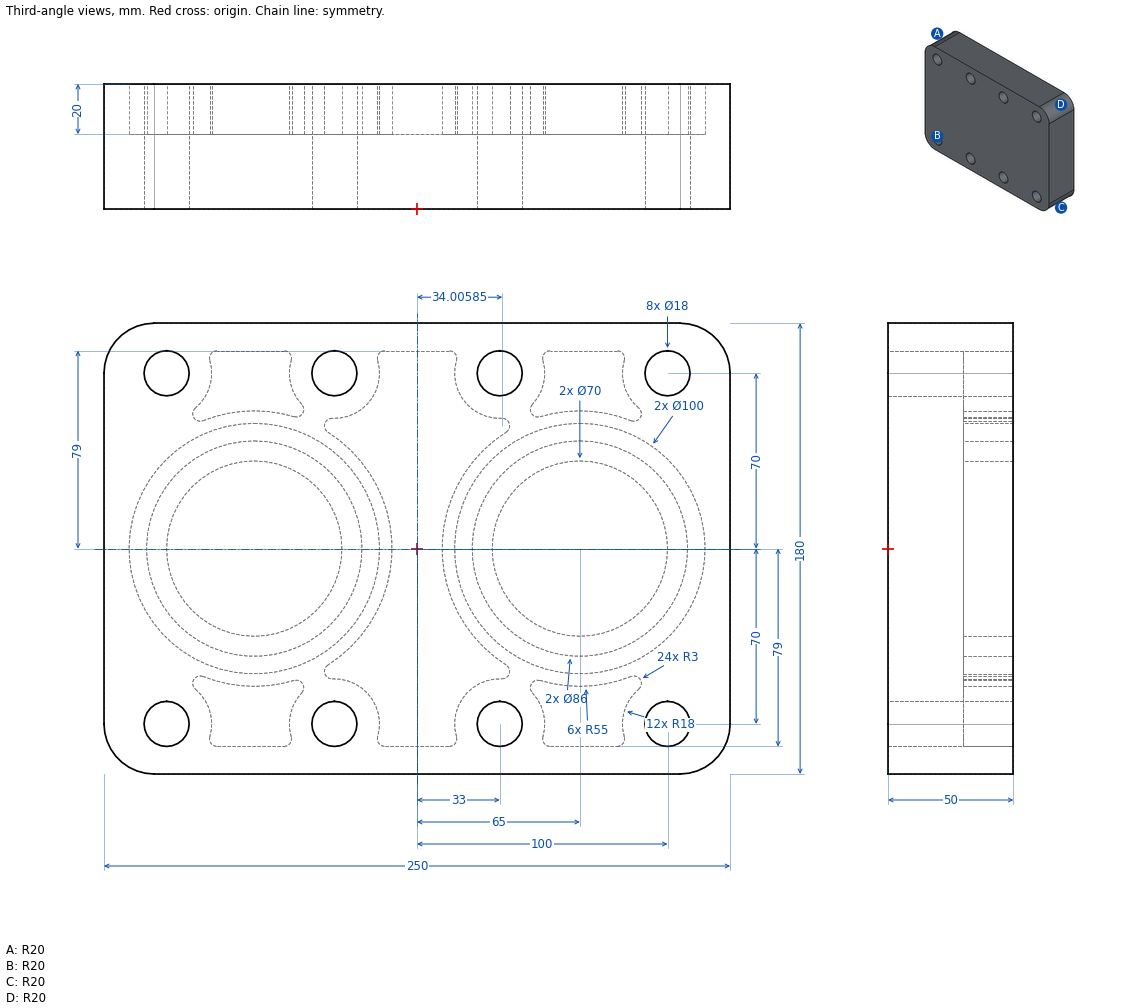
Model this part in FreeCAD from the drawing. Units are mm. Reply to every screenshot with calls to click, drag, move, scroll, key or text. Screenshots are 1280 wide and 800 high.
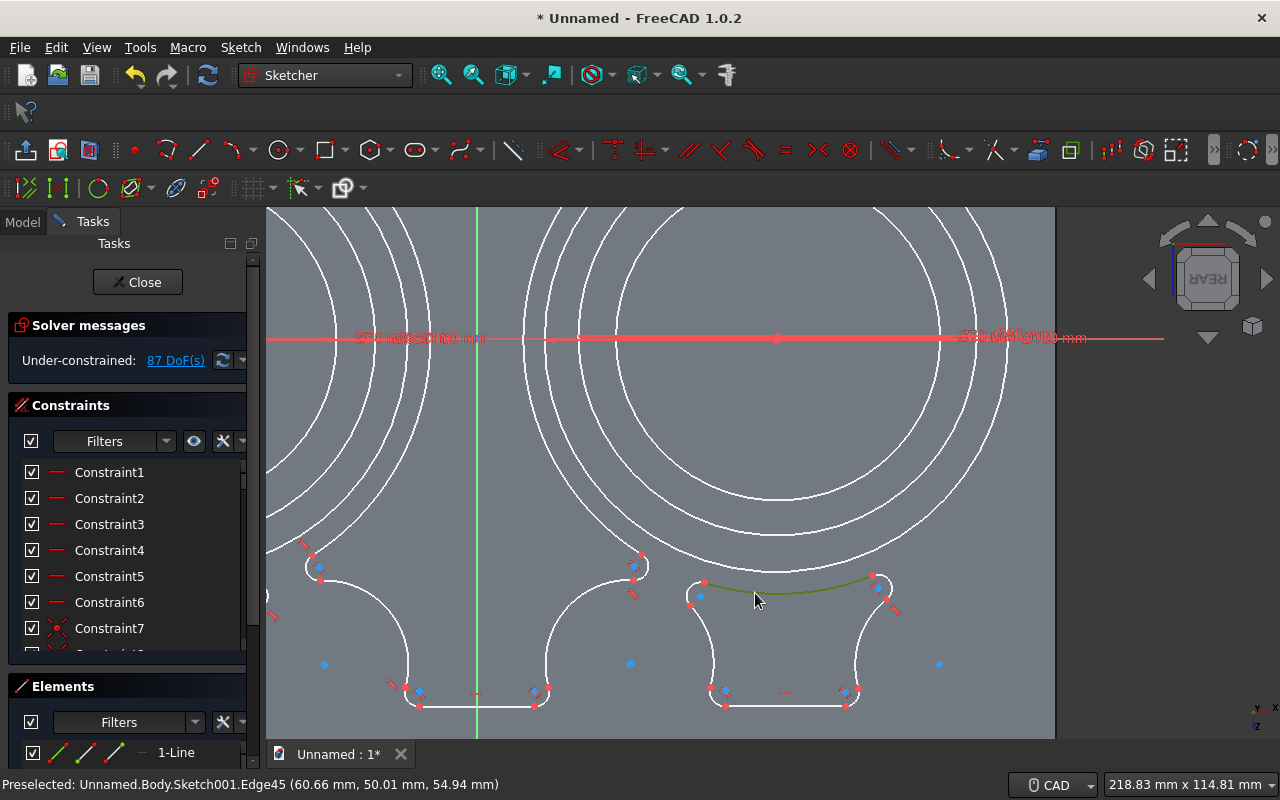
scroll(694, 584, up, 2)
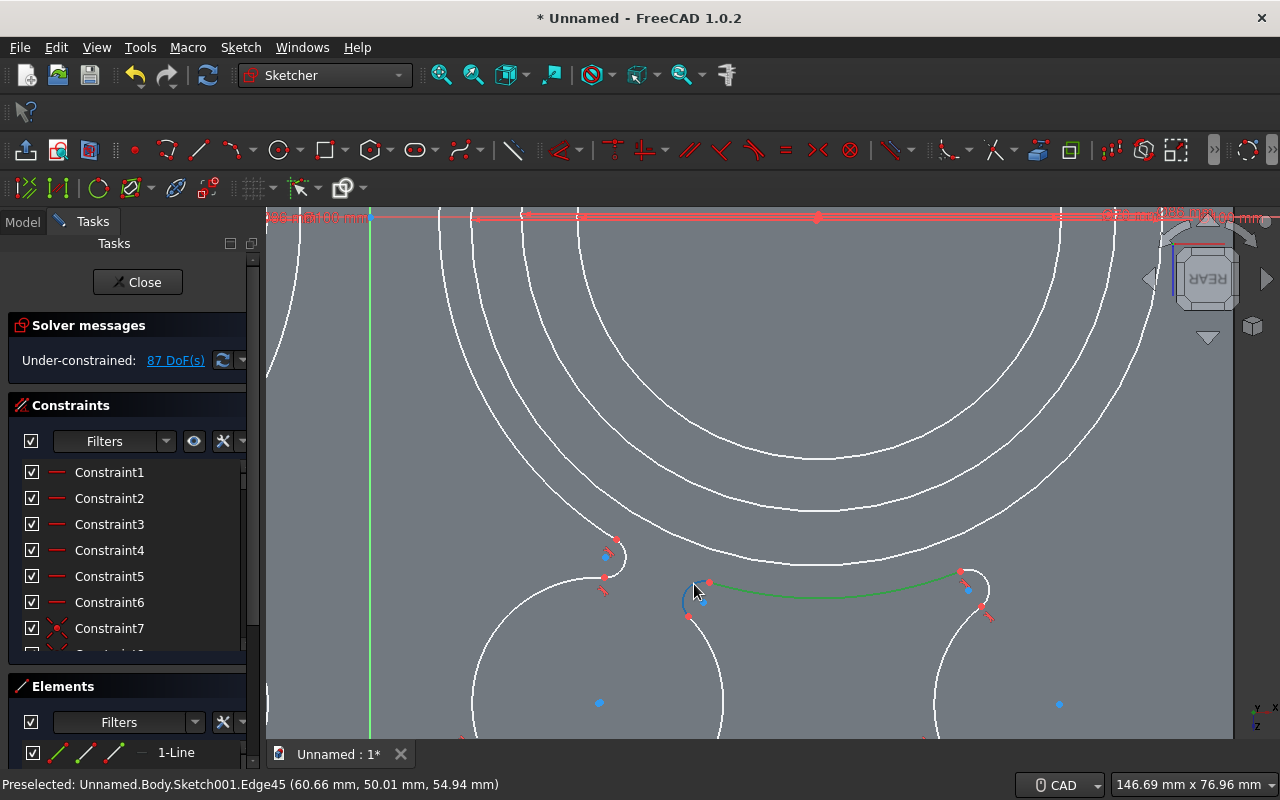
click(693, 584)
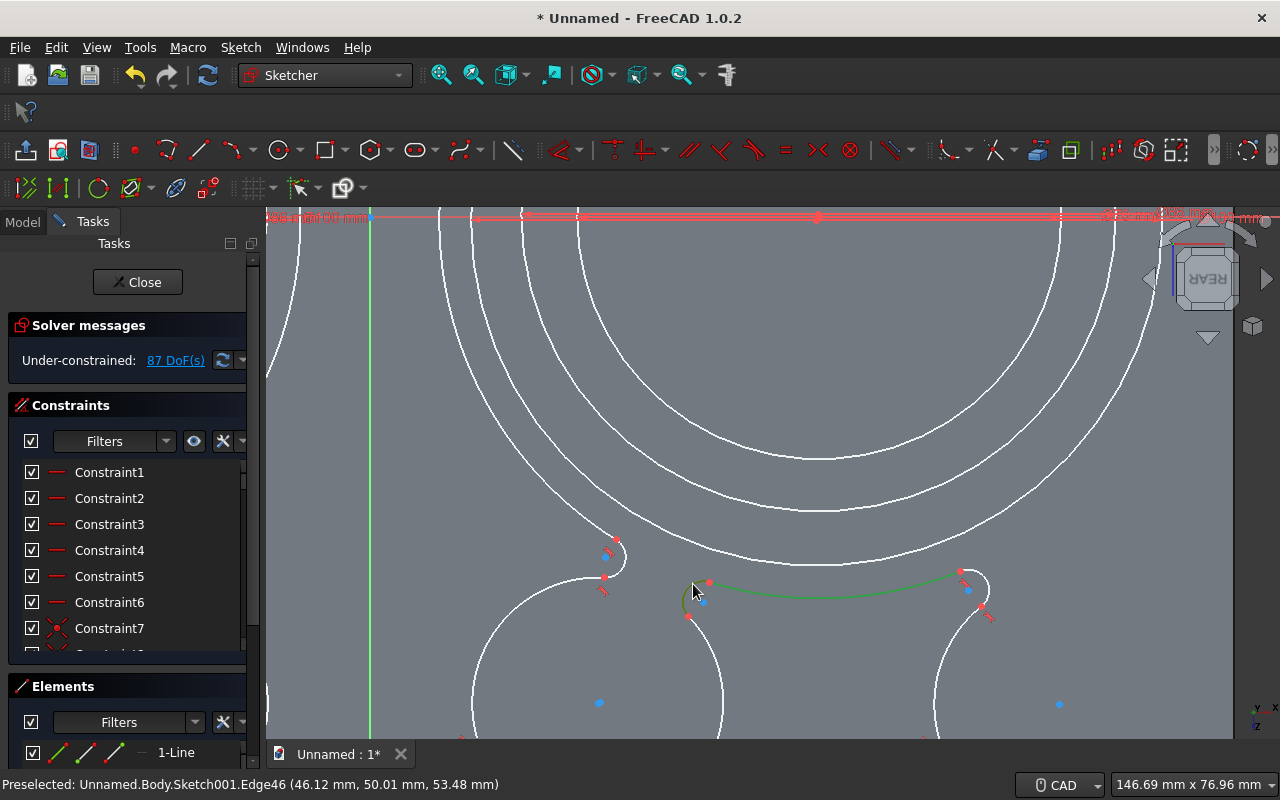
click(754, 150)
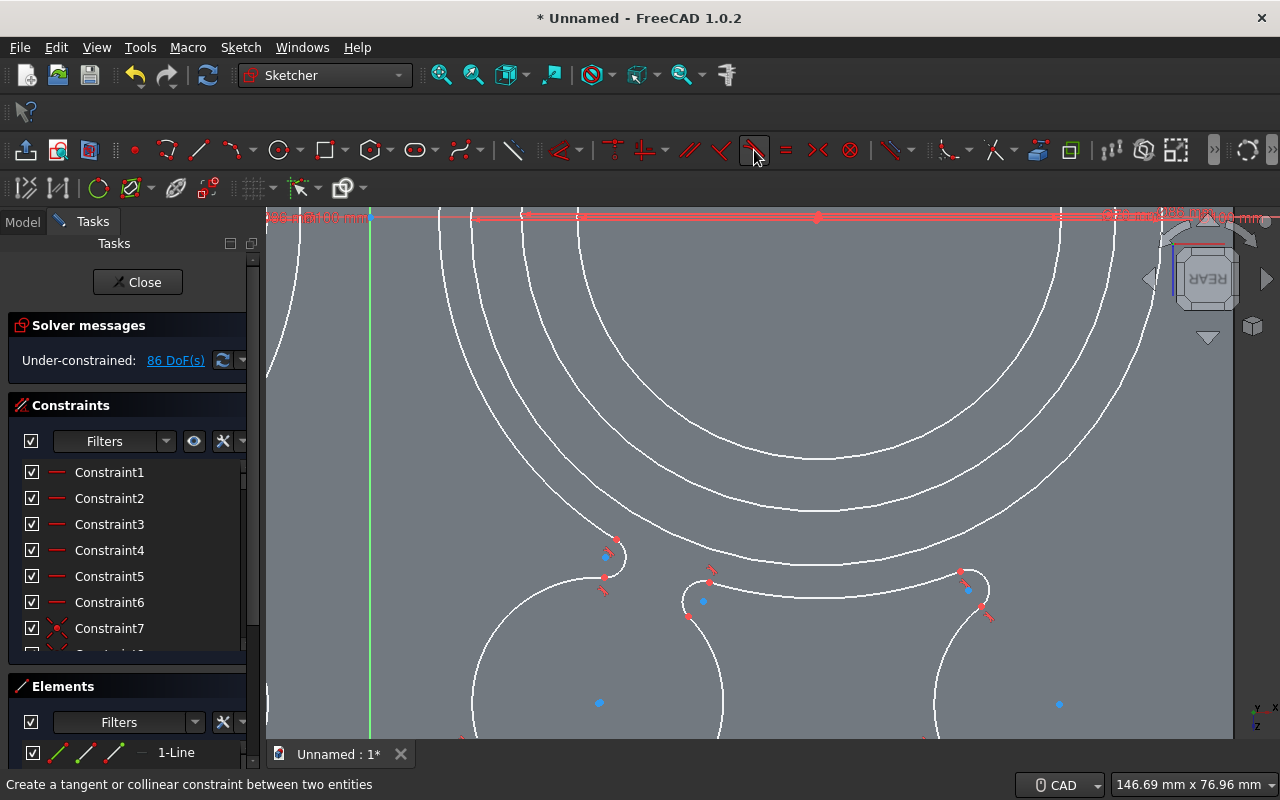
click(693, 584)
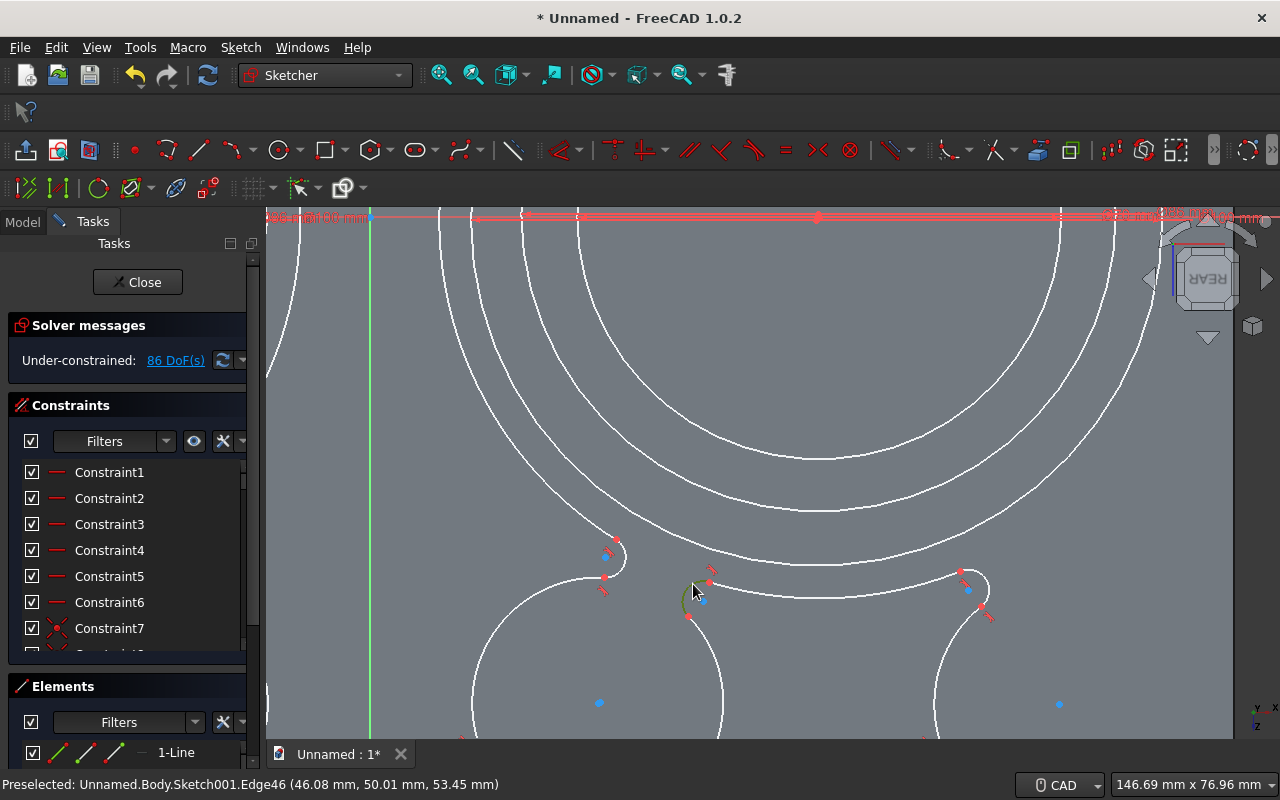
click(723, 699)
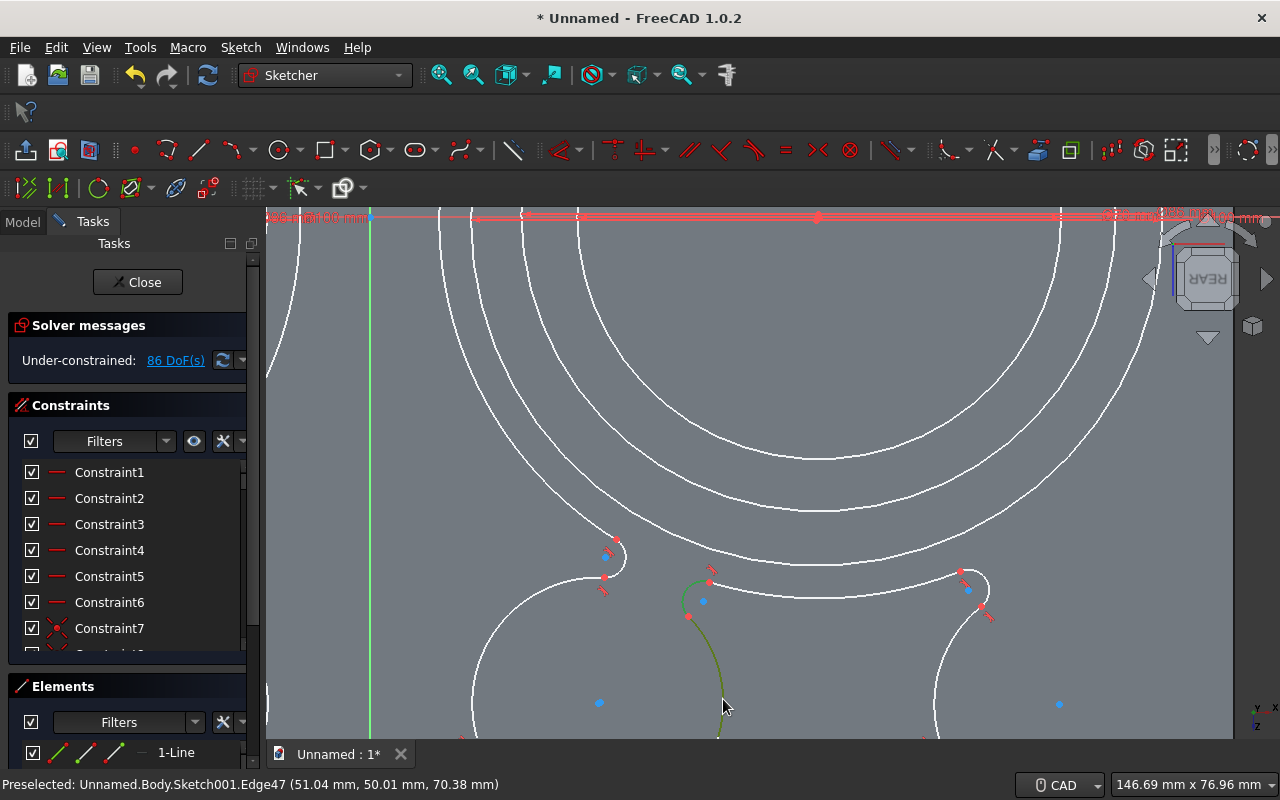
click(754, 150)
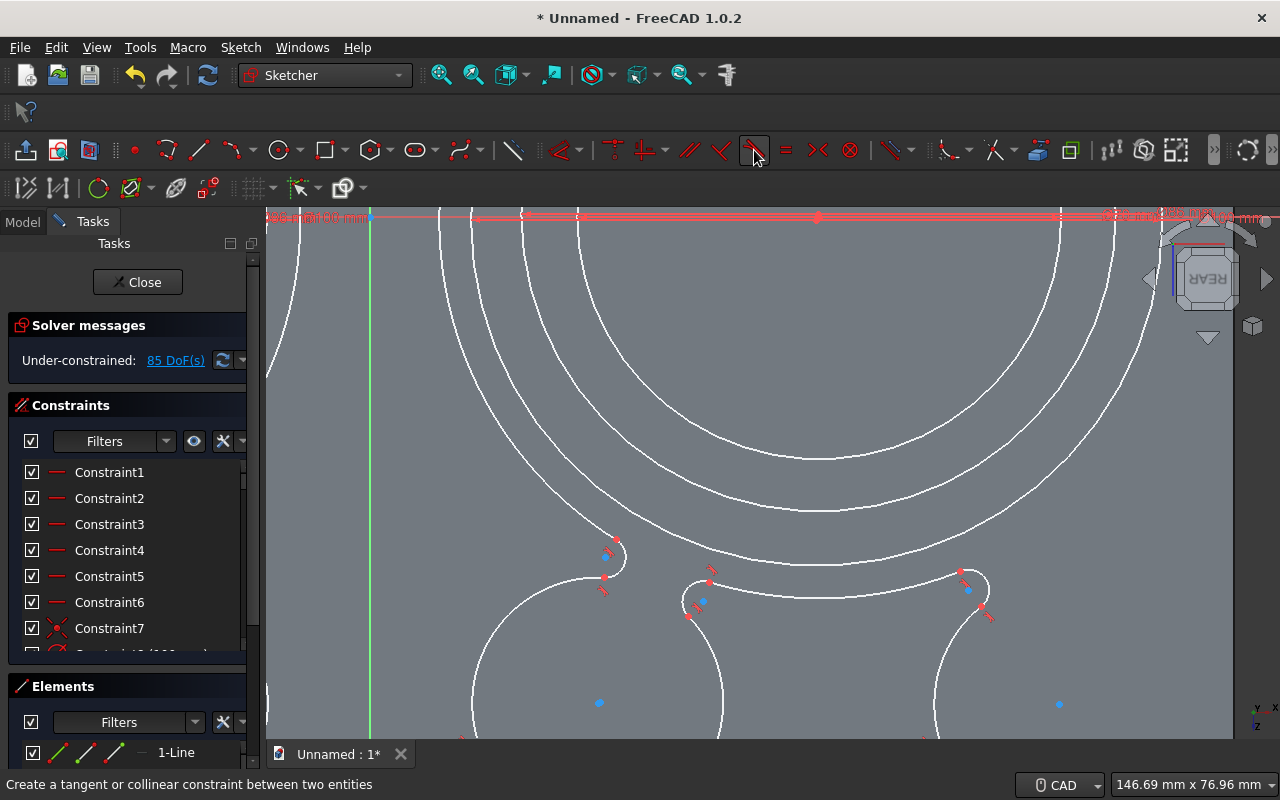
click(723, 699)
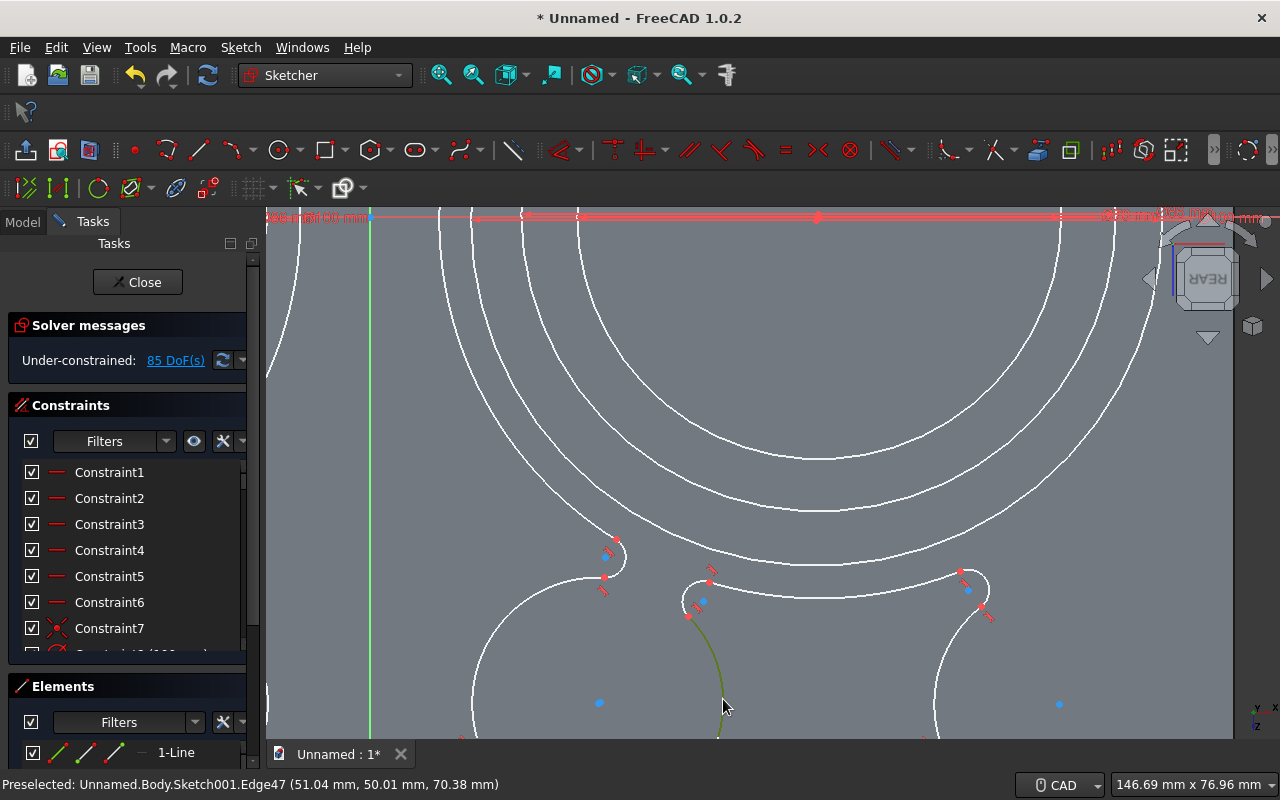
scroll(849, 583, down, 6)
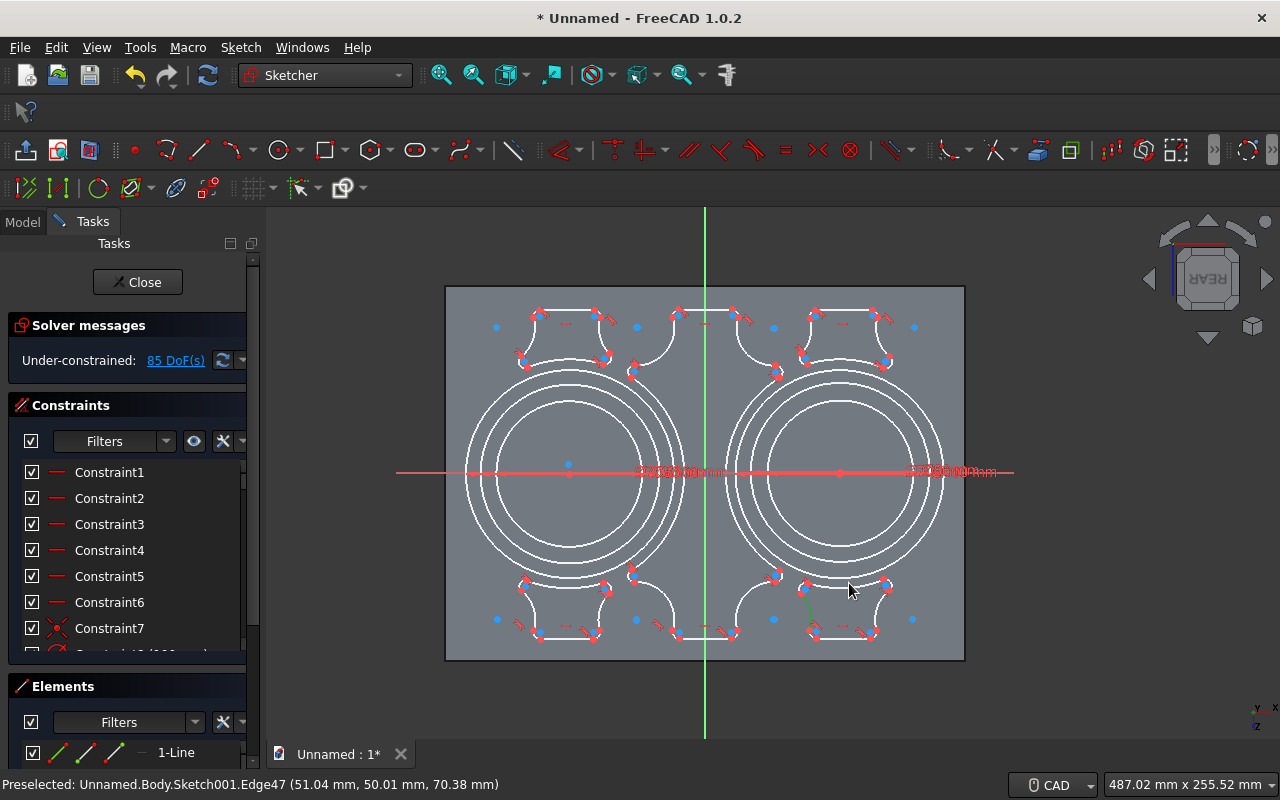
scroll(810, 634, up, 7)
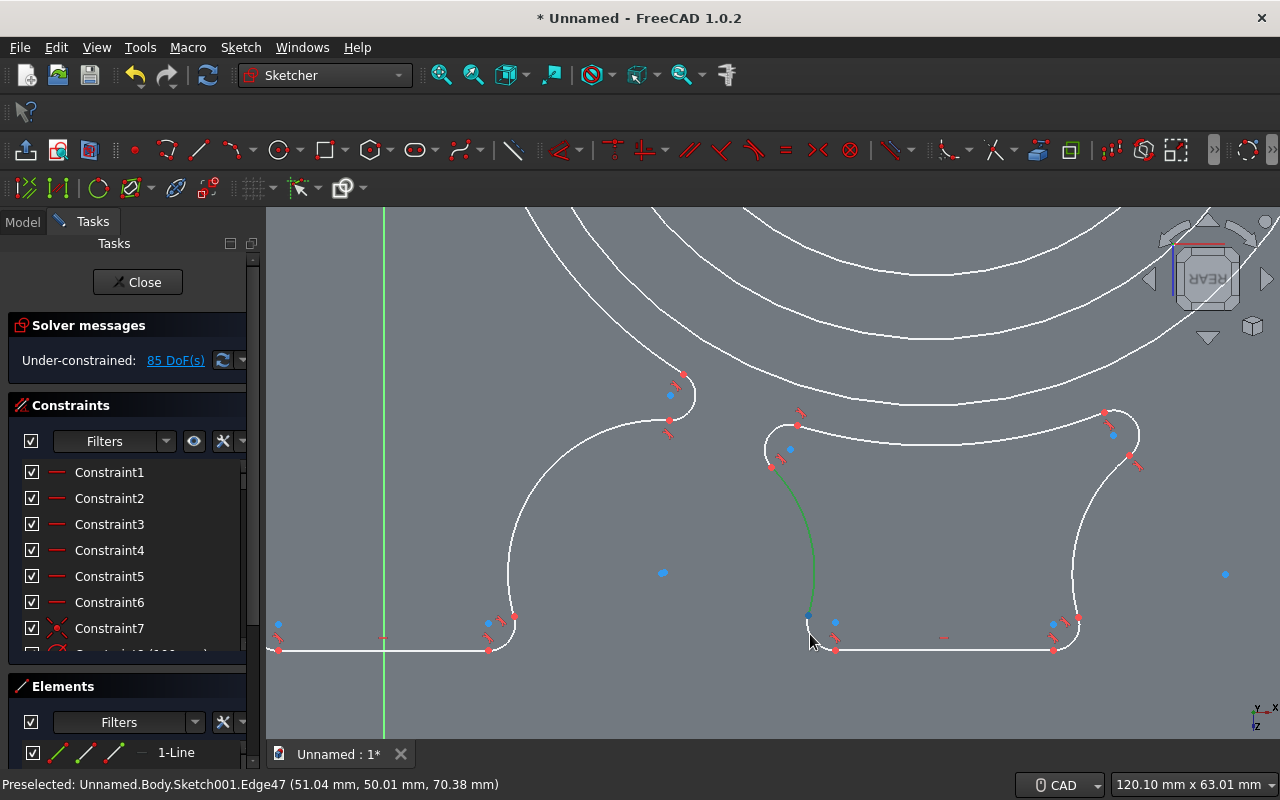
click(808, 630)